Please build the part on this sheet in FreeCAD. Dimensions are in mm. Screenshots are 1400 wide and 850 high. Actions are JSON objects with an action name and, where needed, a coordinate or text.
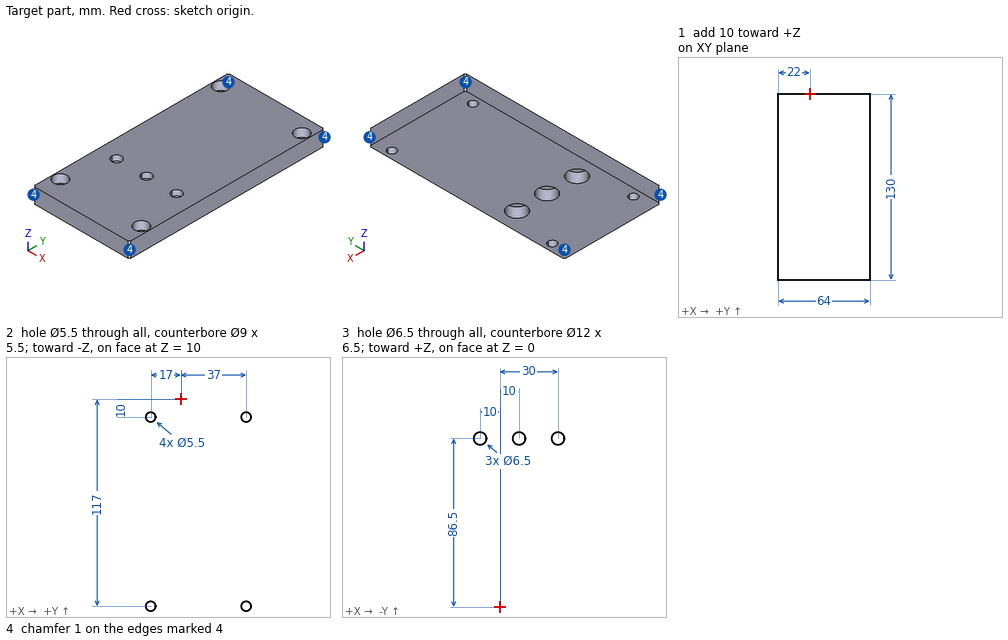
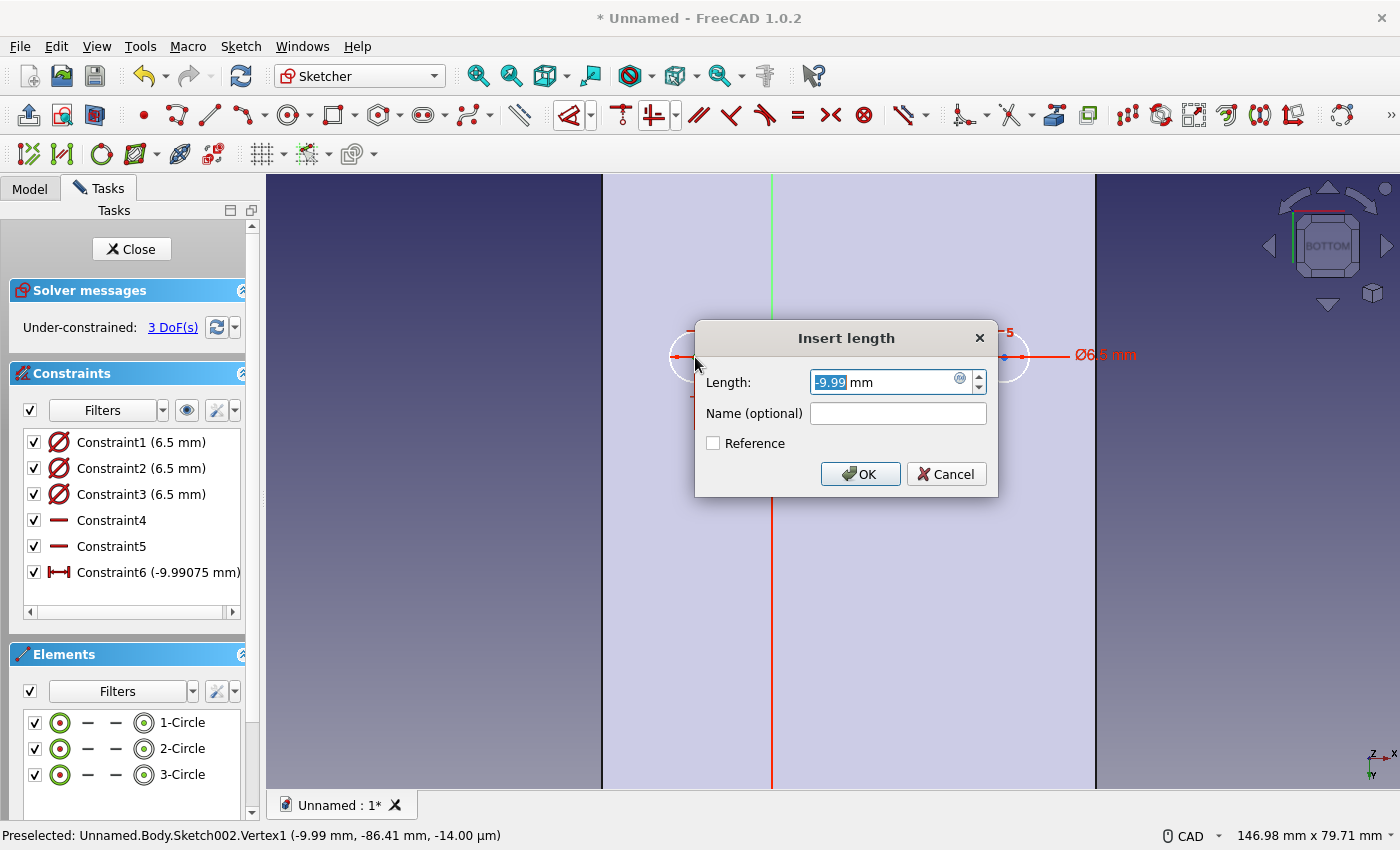
{"action": "type", "text": "-10"}
{"action": "key", "text": "Return"}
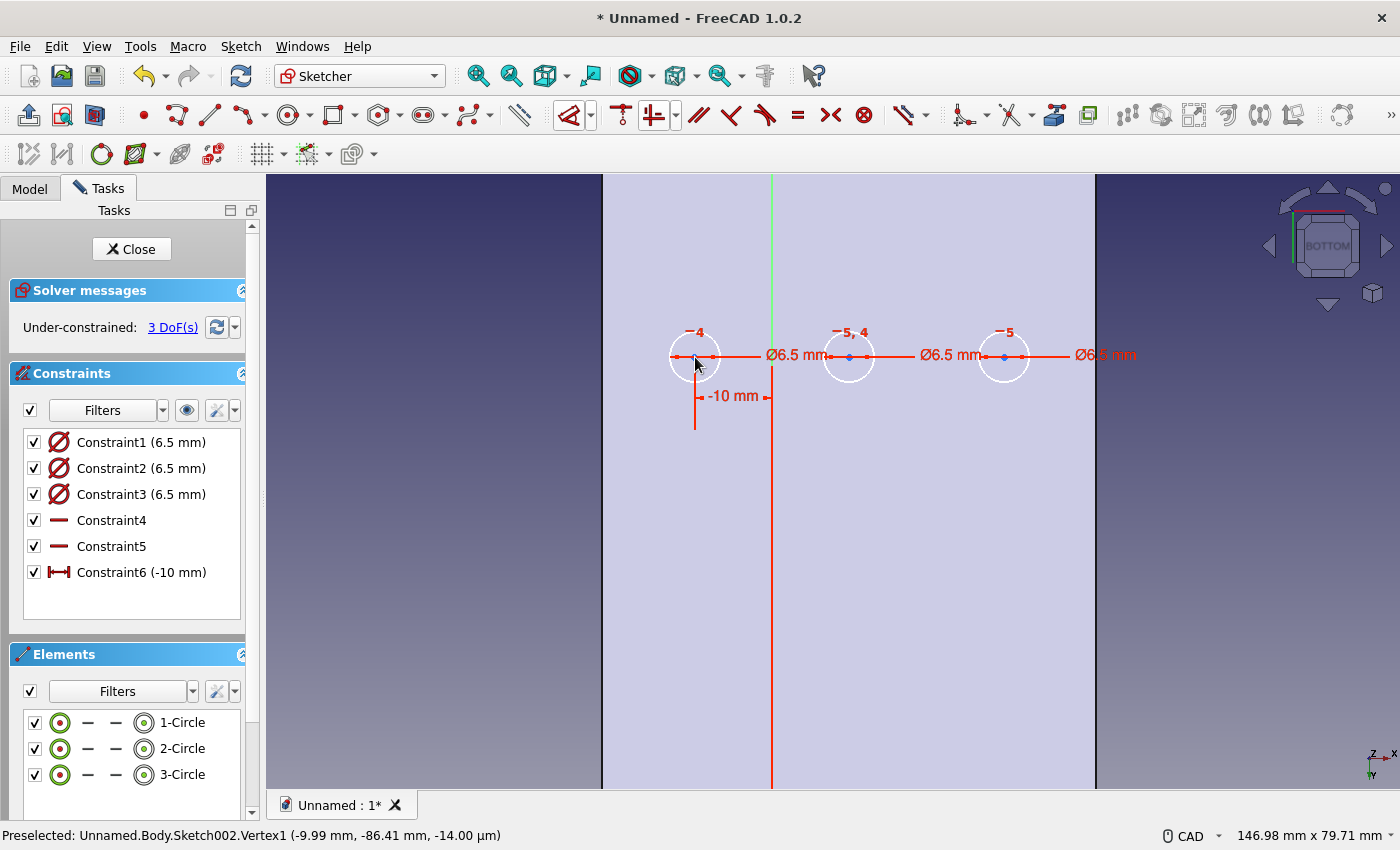
{"action": "left_click", "coordinate": [849, 357]}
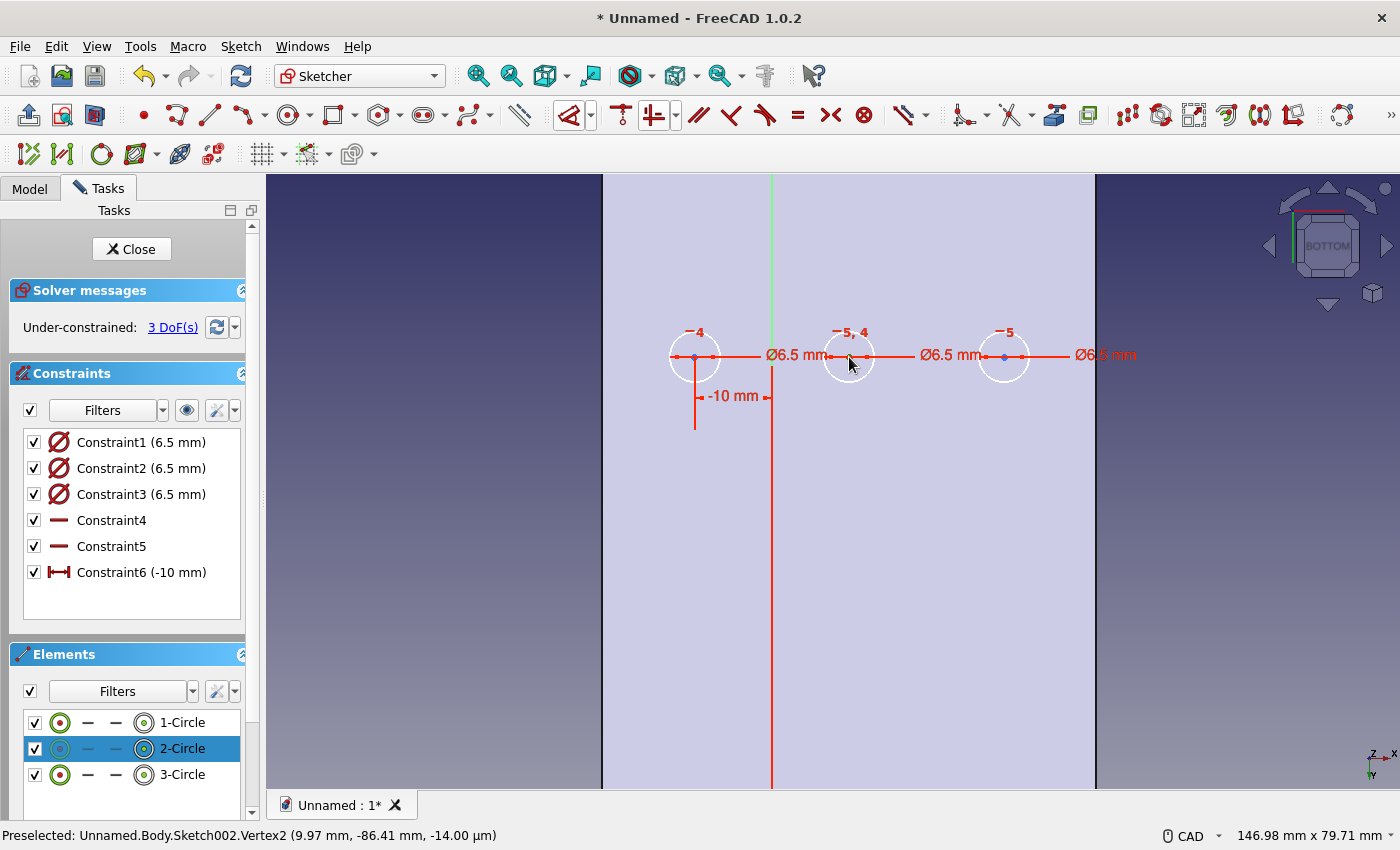
{"action": "key", "text": "l"}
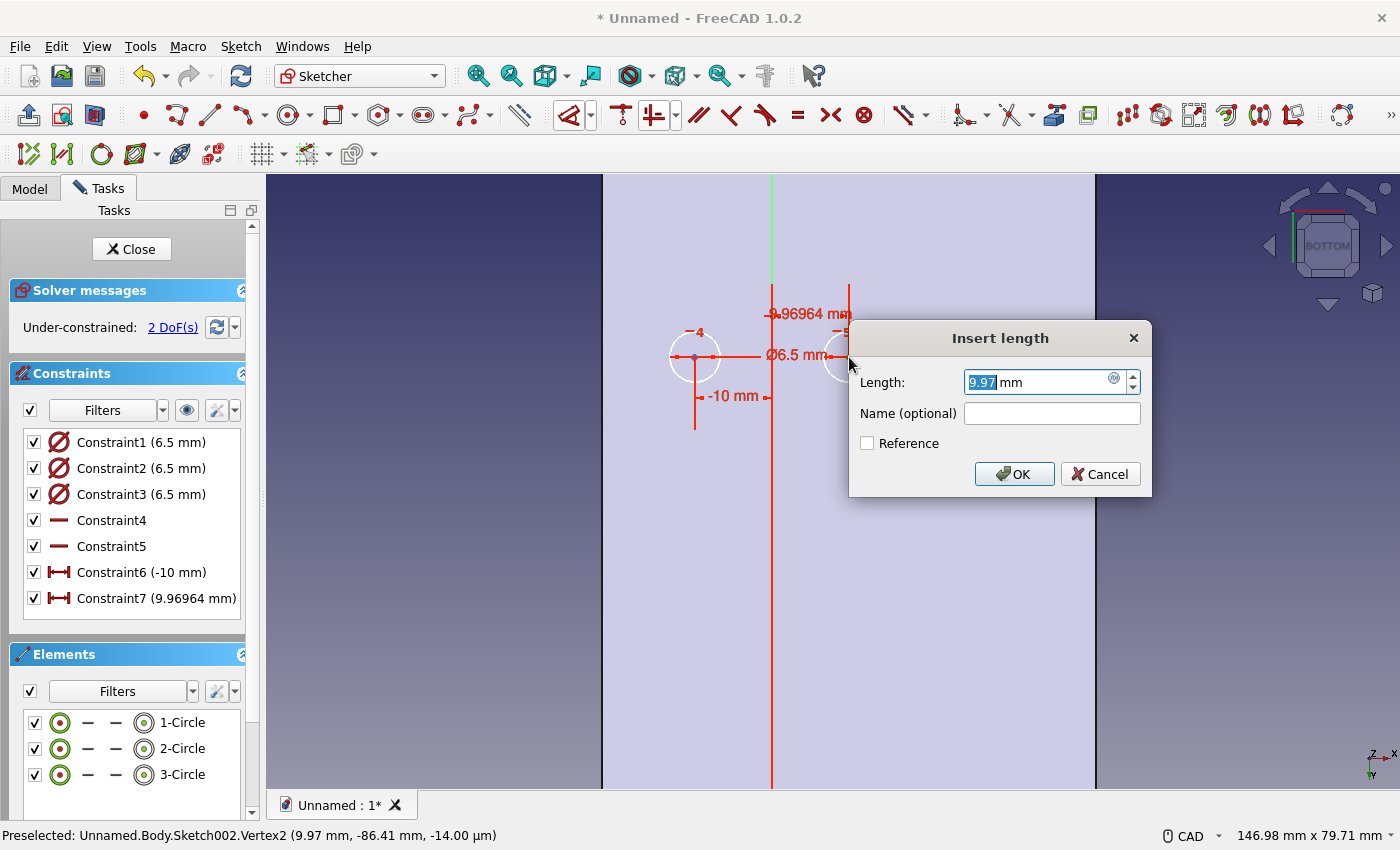
{"action": "type", "text": "10"}
{"action": "key", "text": "Return"}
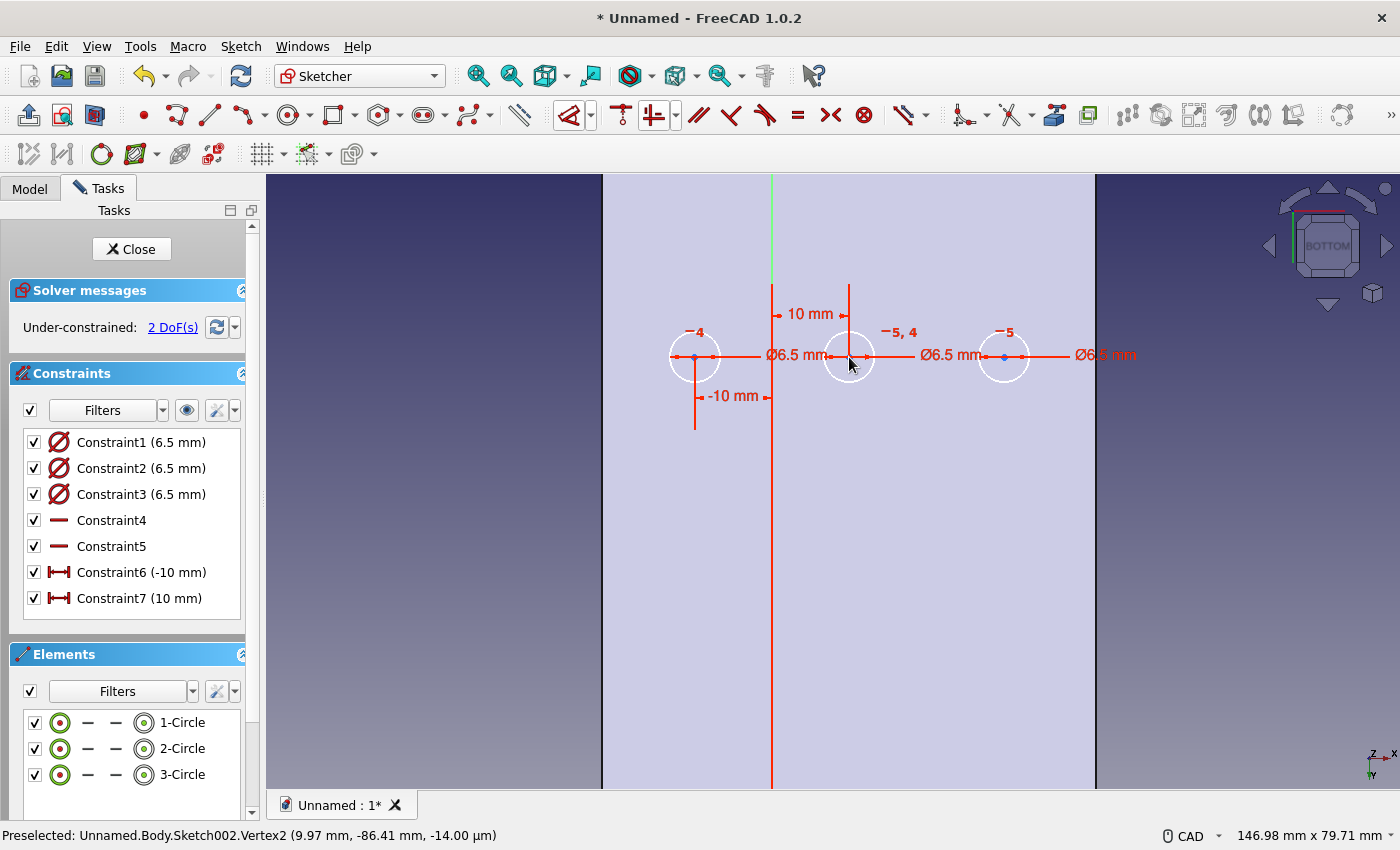
{"action": "left_click", "coordinate": [1004, 357]}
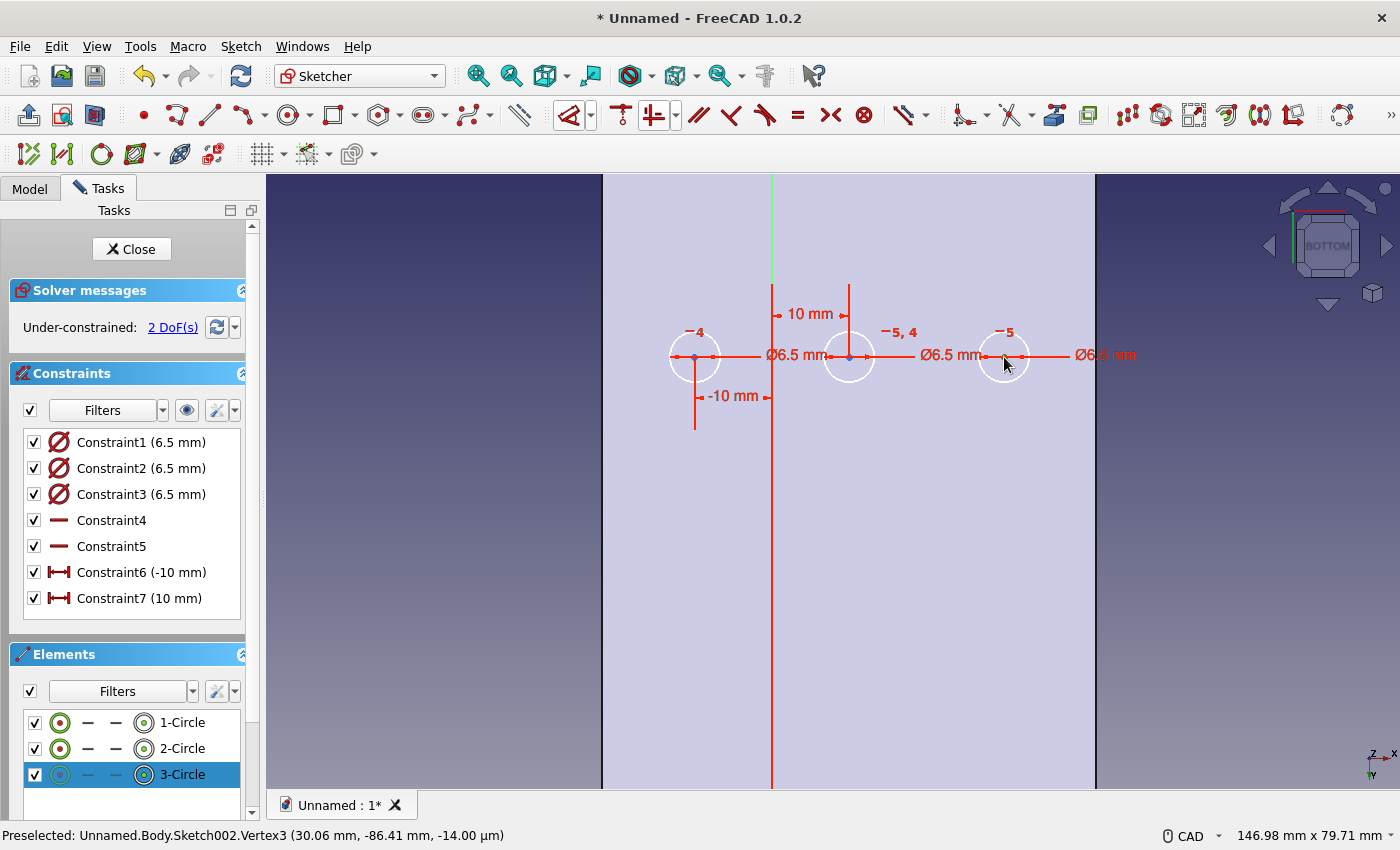
{"action": "key", "text": "l"}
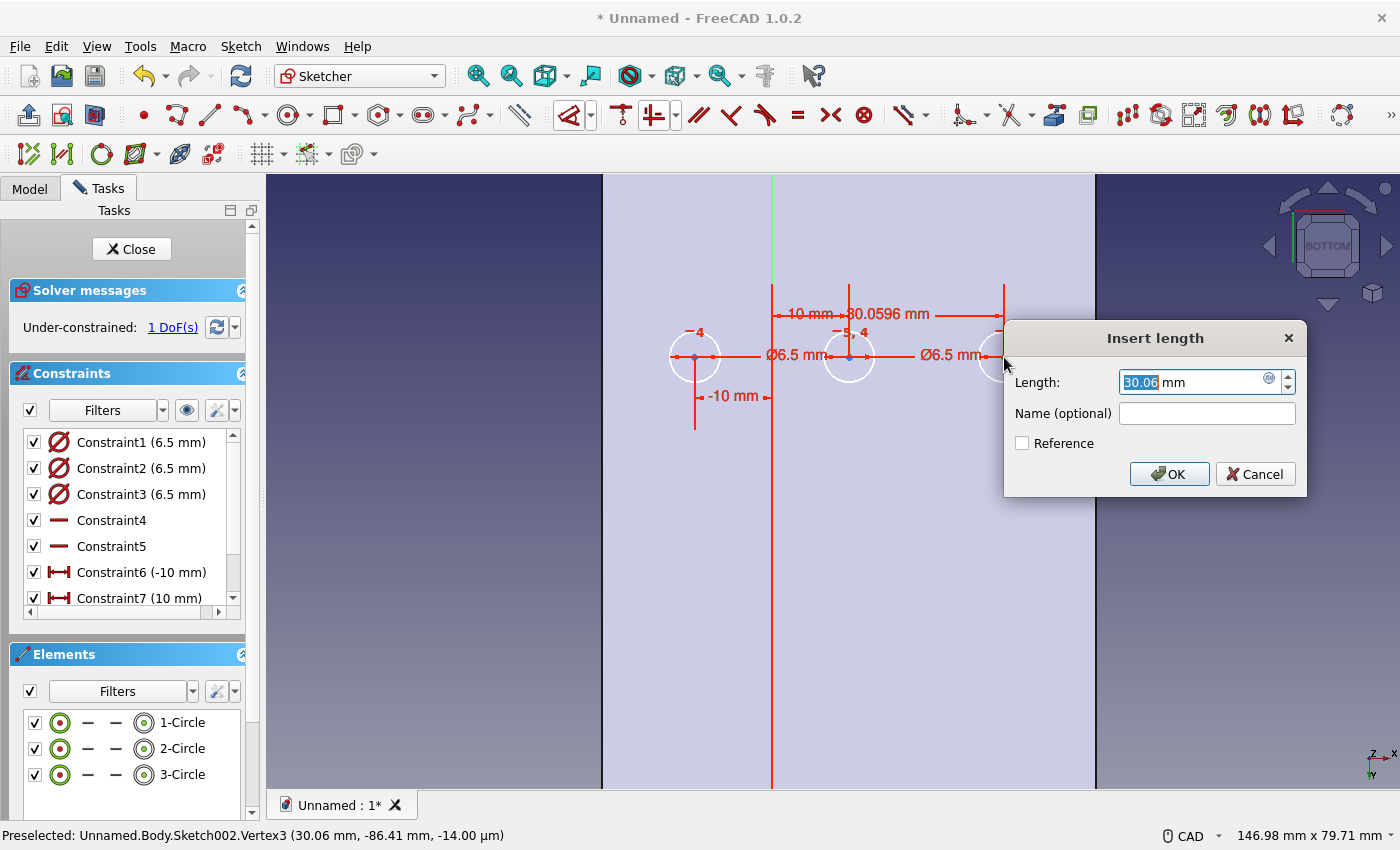
{"action": "type", "text": "30"}
{"action": "key", "text": "Return"}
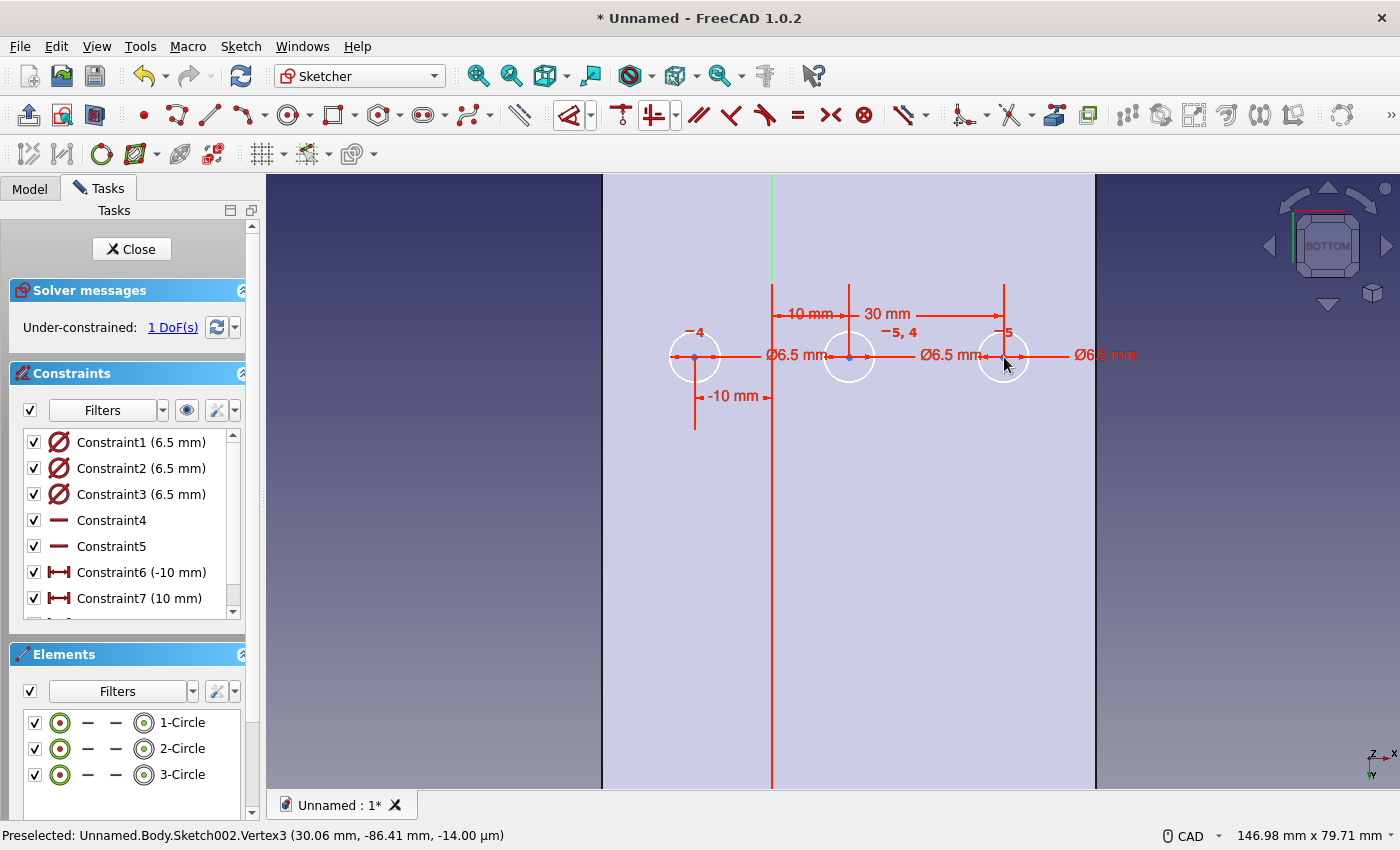
{"action": "left_click", "coordinate": [695, 357]}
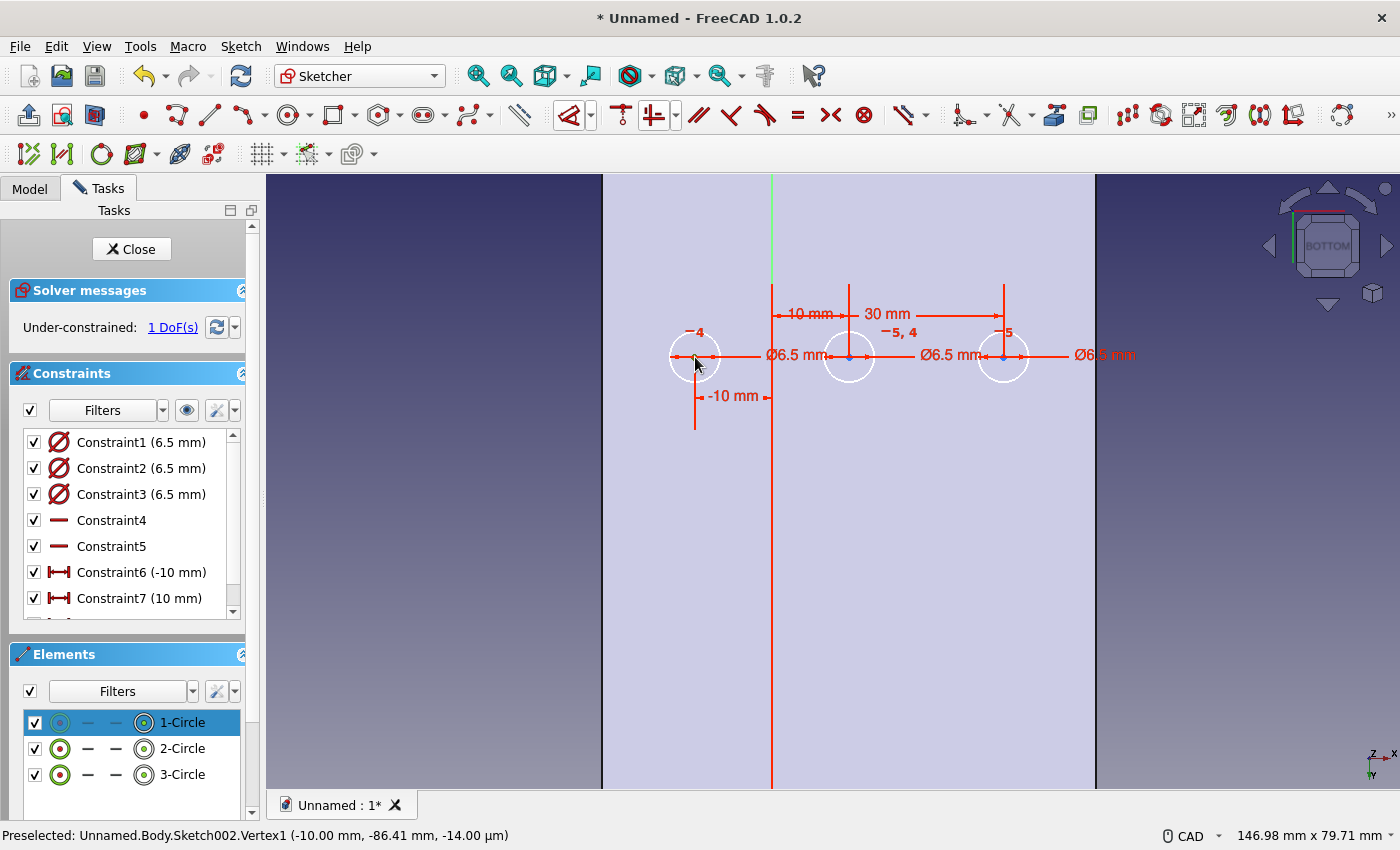
{"action": "key", "text": "i"}